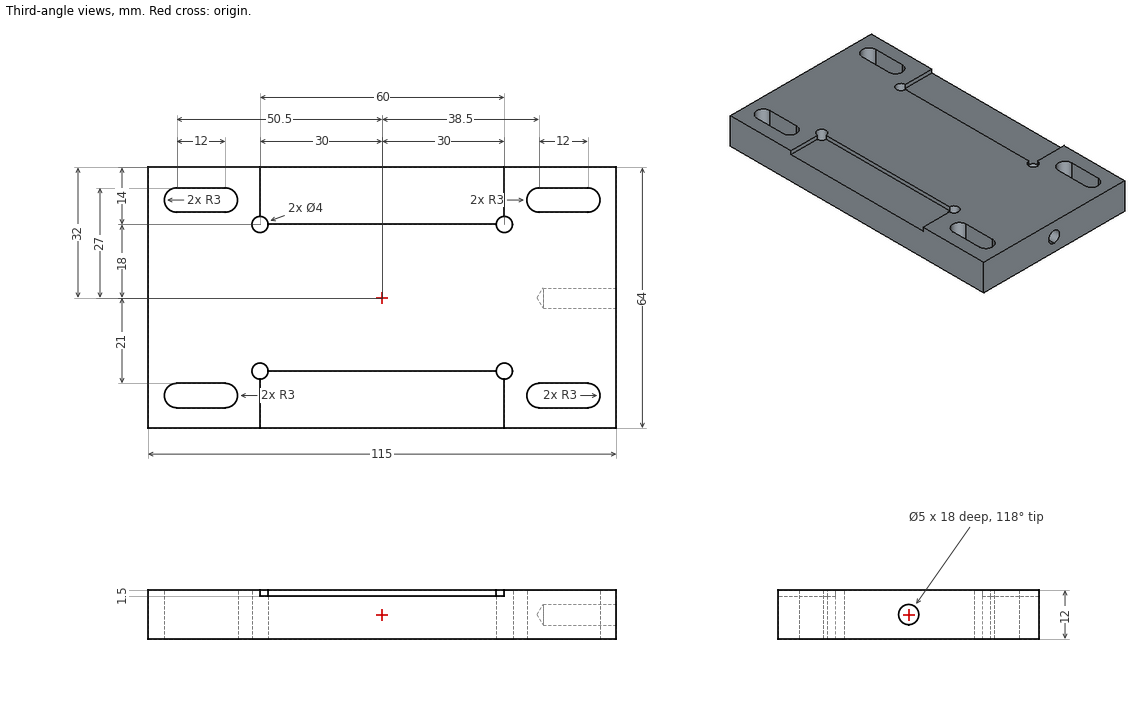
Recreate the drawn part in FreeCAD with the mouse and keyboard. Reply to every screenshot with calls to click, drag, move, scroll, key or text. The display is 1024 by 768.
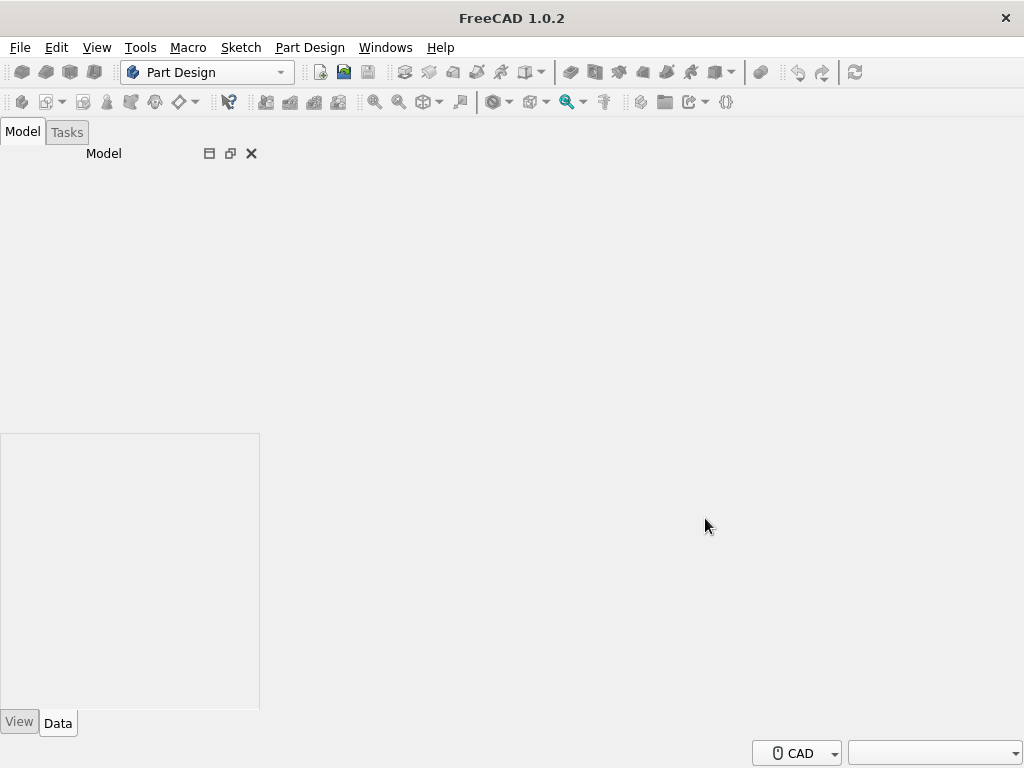
click(320, 72)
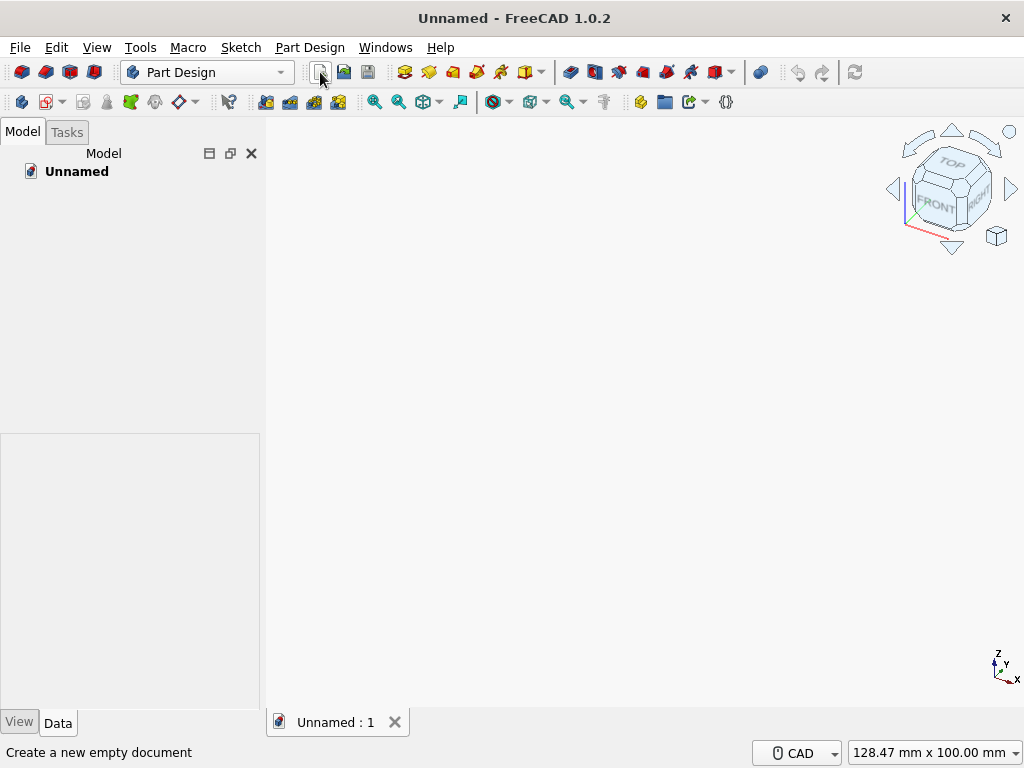
click(46, 102)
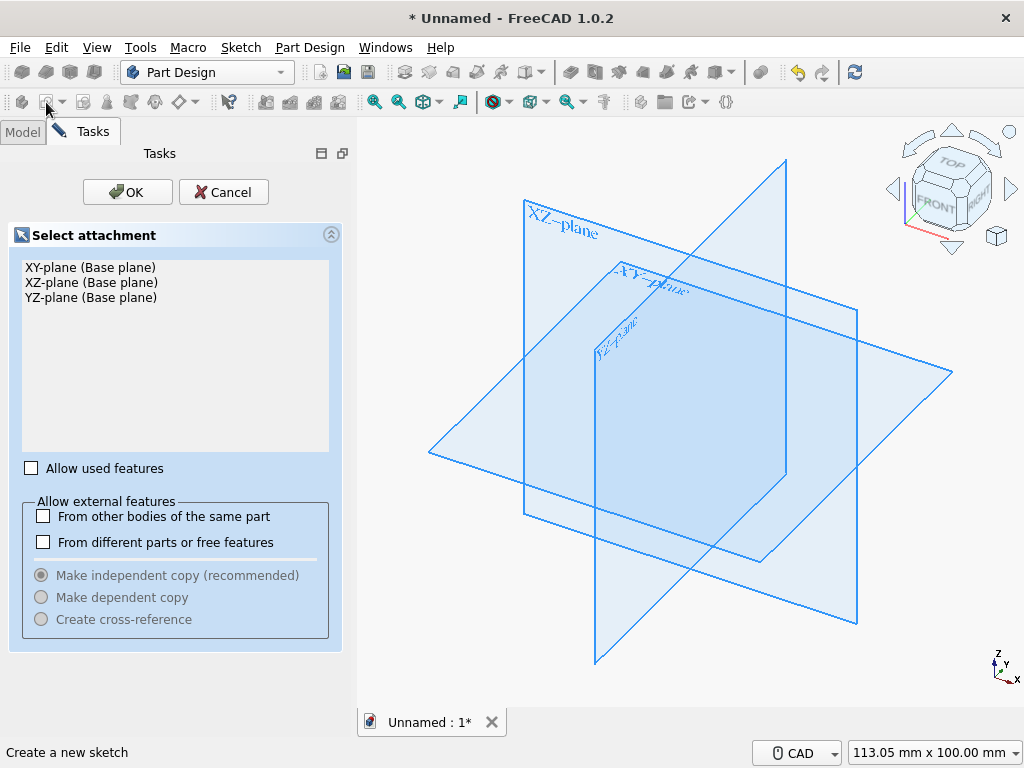
click(82, 268)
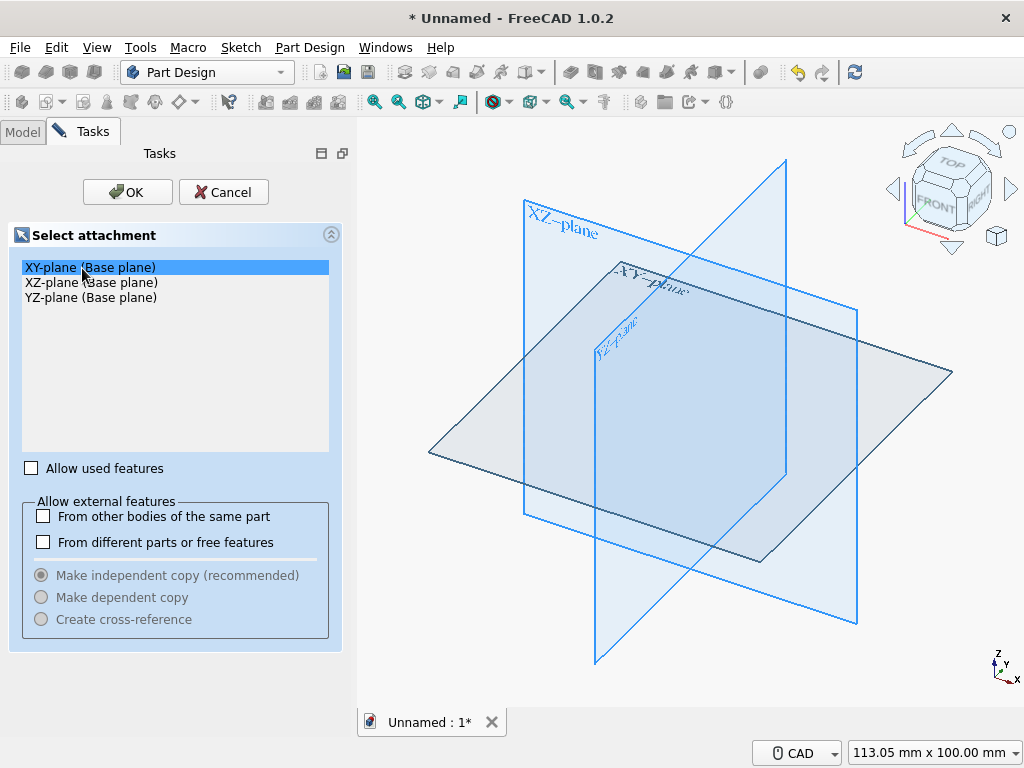
click(128, 192)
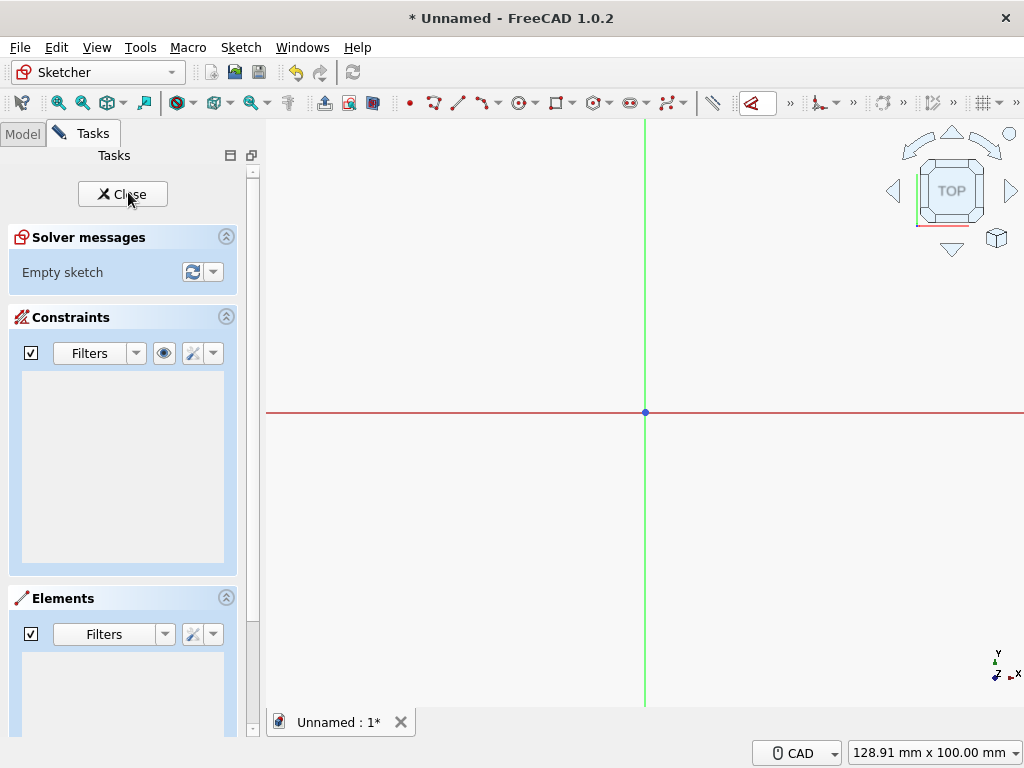
scroll(493, 413, down, 3)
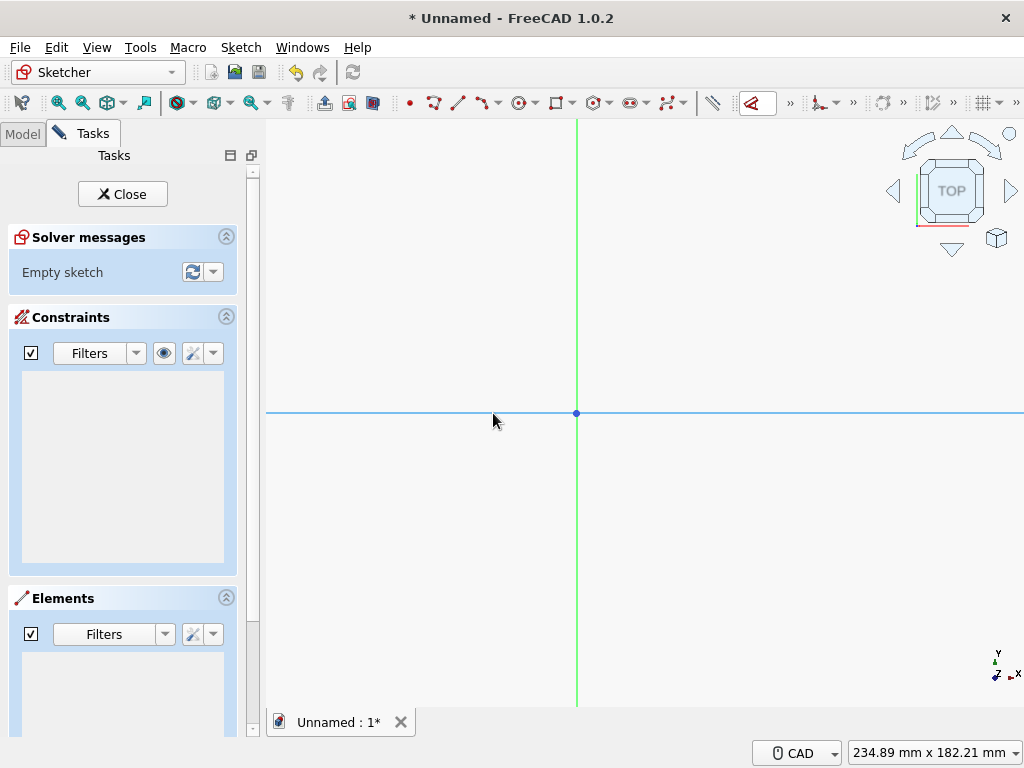
click(574, 104)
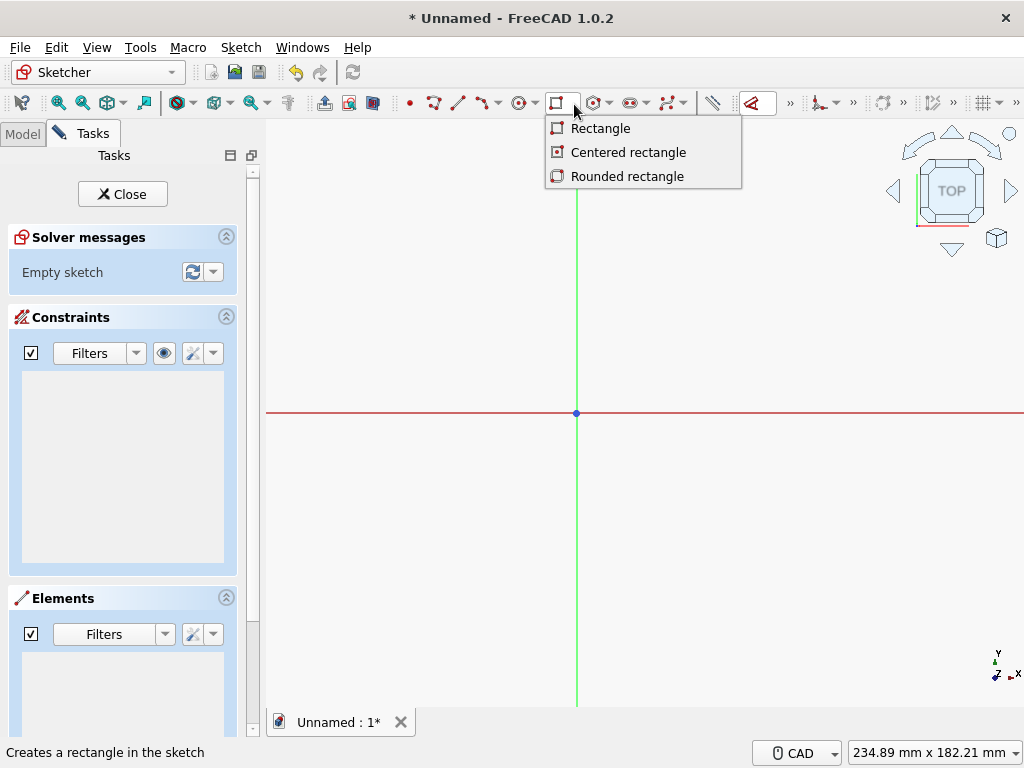
click(644, 152)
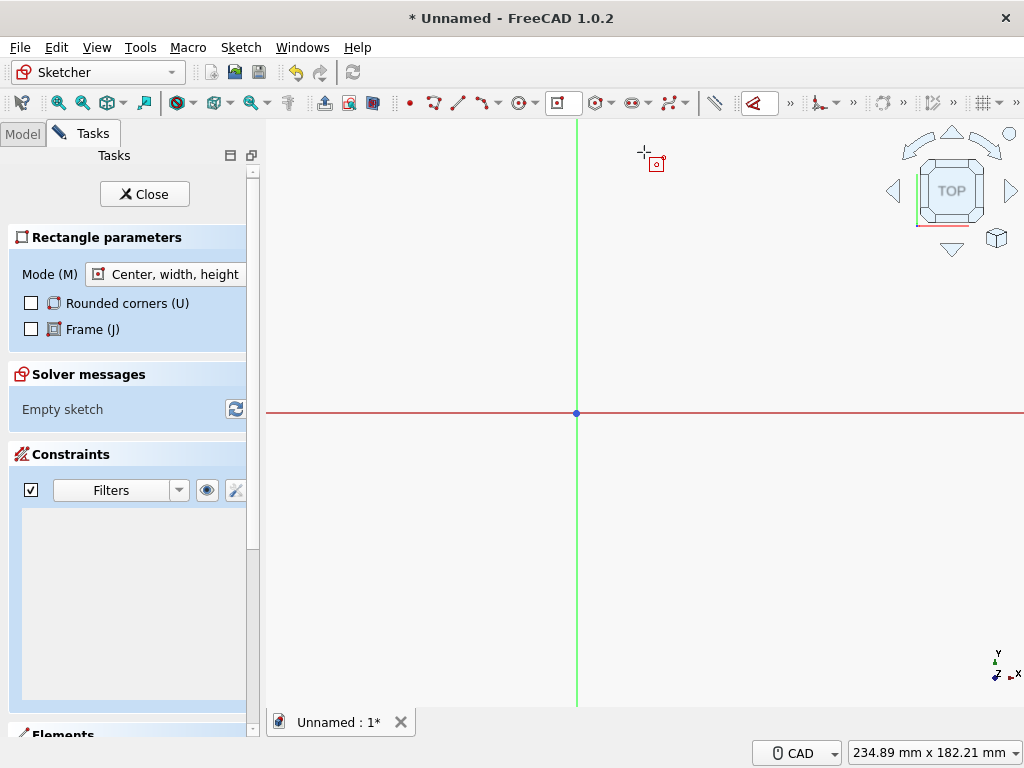
click(577, 413)
click(762, 310)
key(Escape)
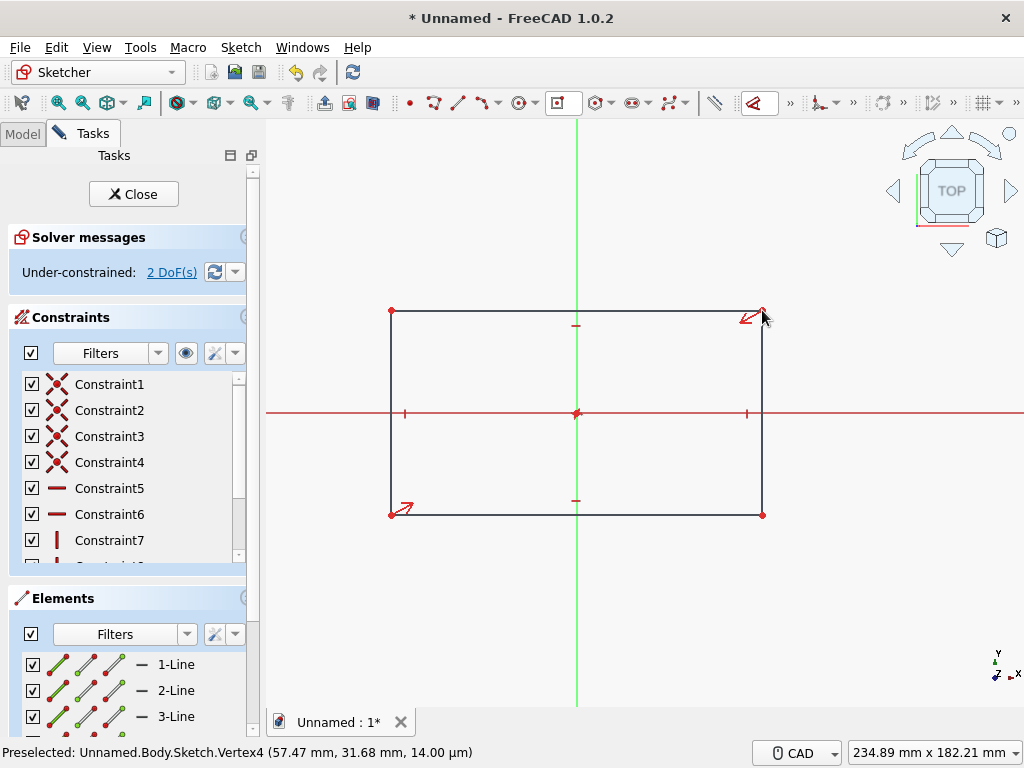
click(762, 454)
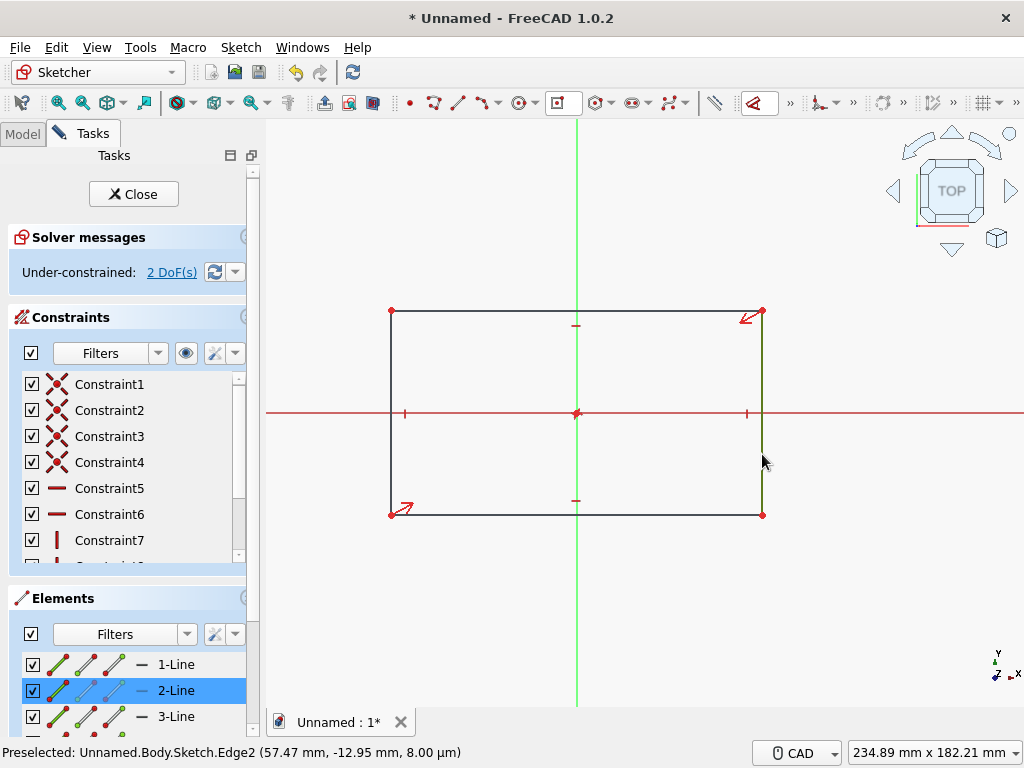
click(772, 104)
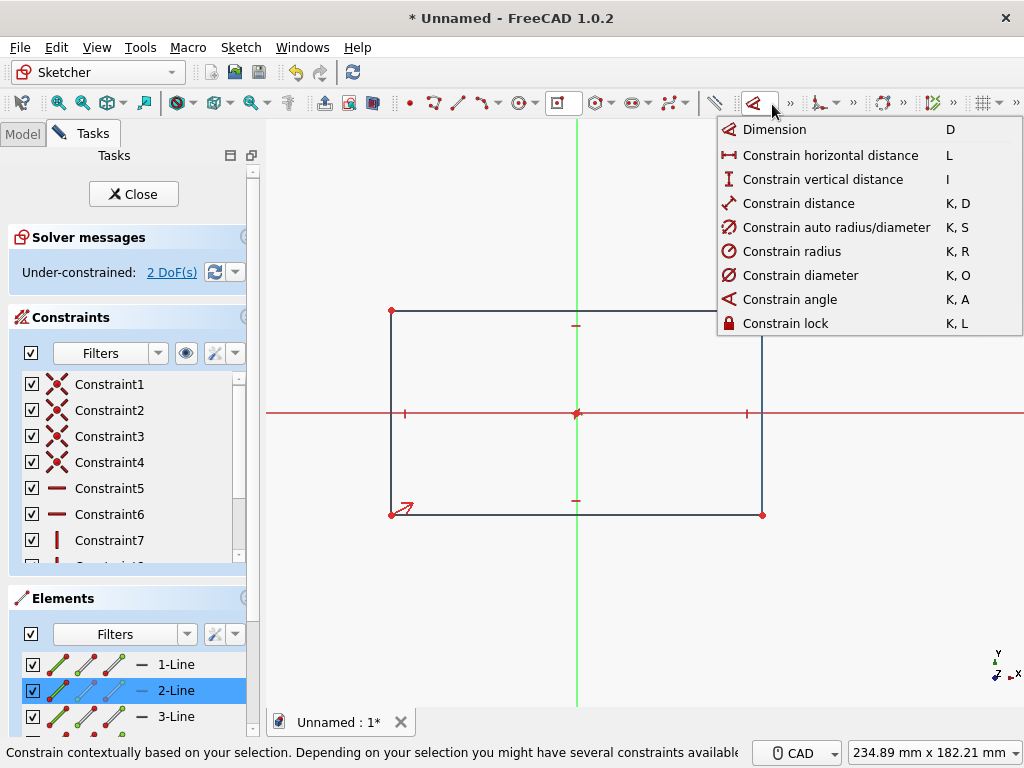
click(870, 179)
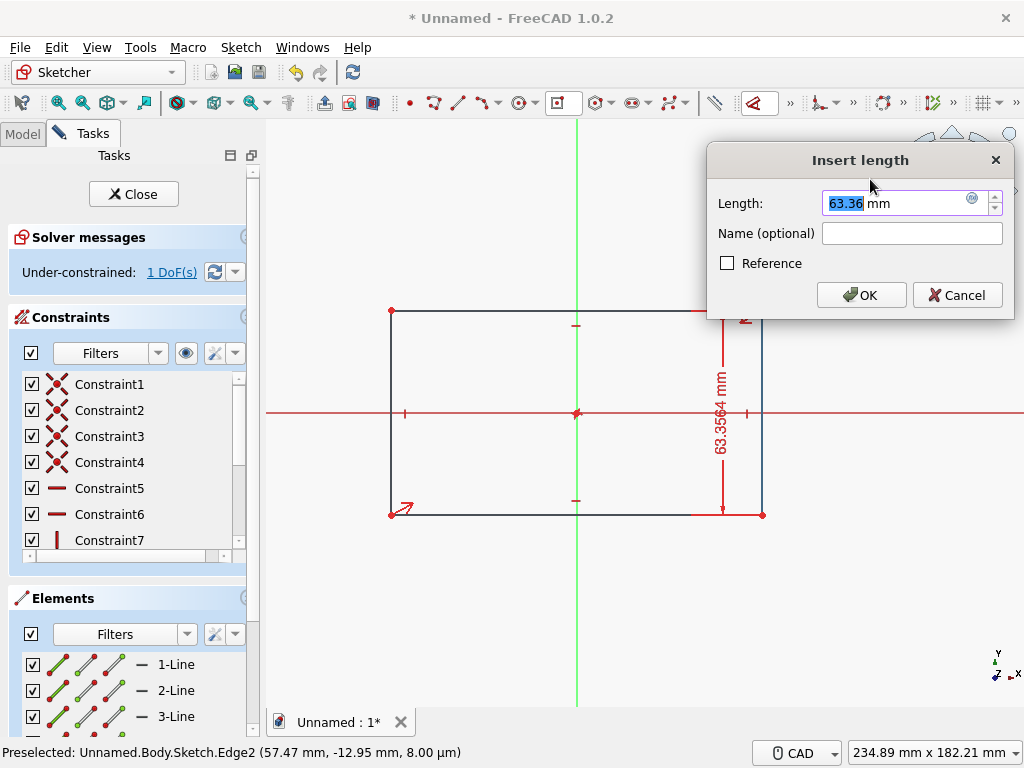
text(64)
key(Return)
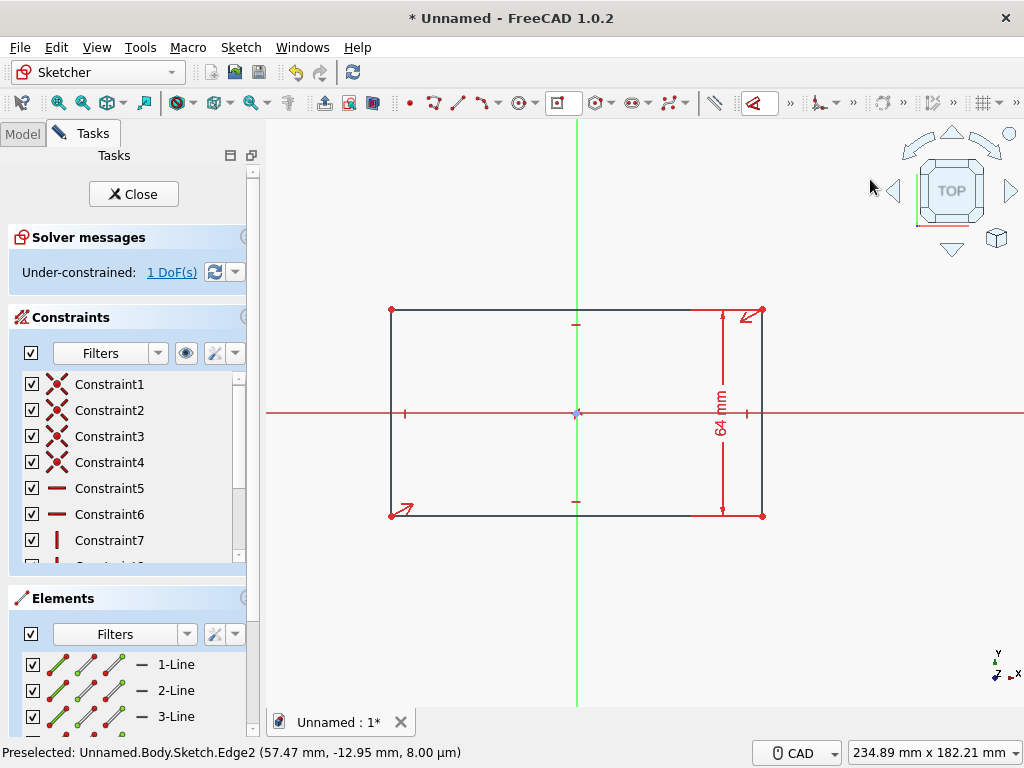
click(502, 516)